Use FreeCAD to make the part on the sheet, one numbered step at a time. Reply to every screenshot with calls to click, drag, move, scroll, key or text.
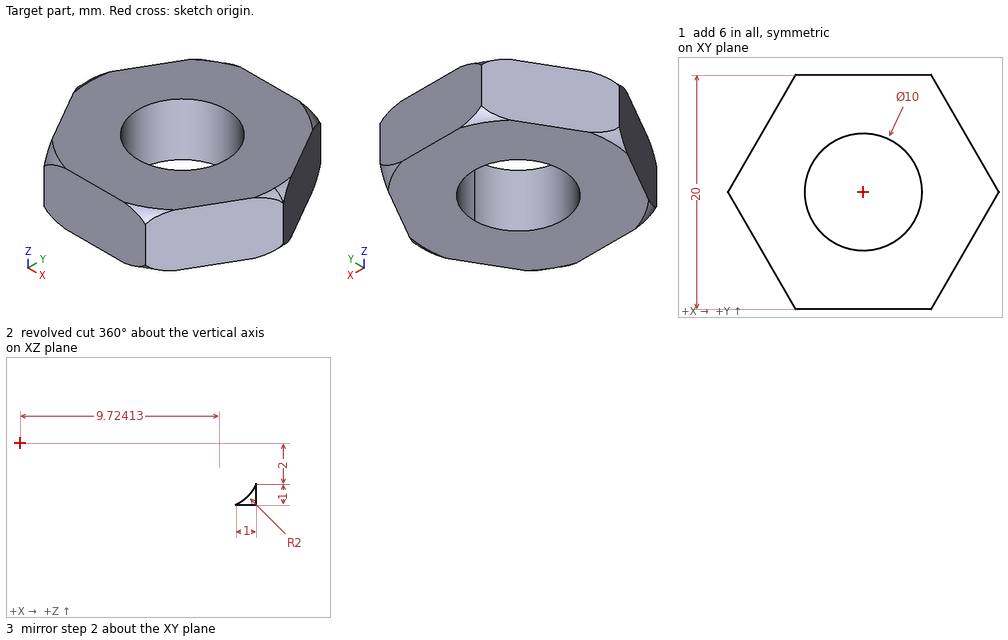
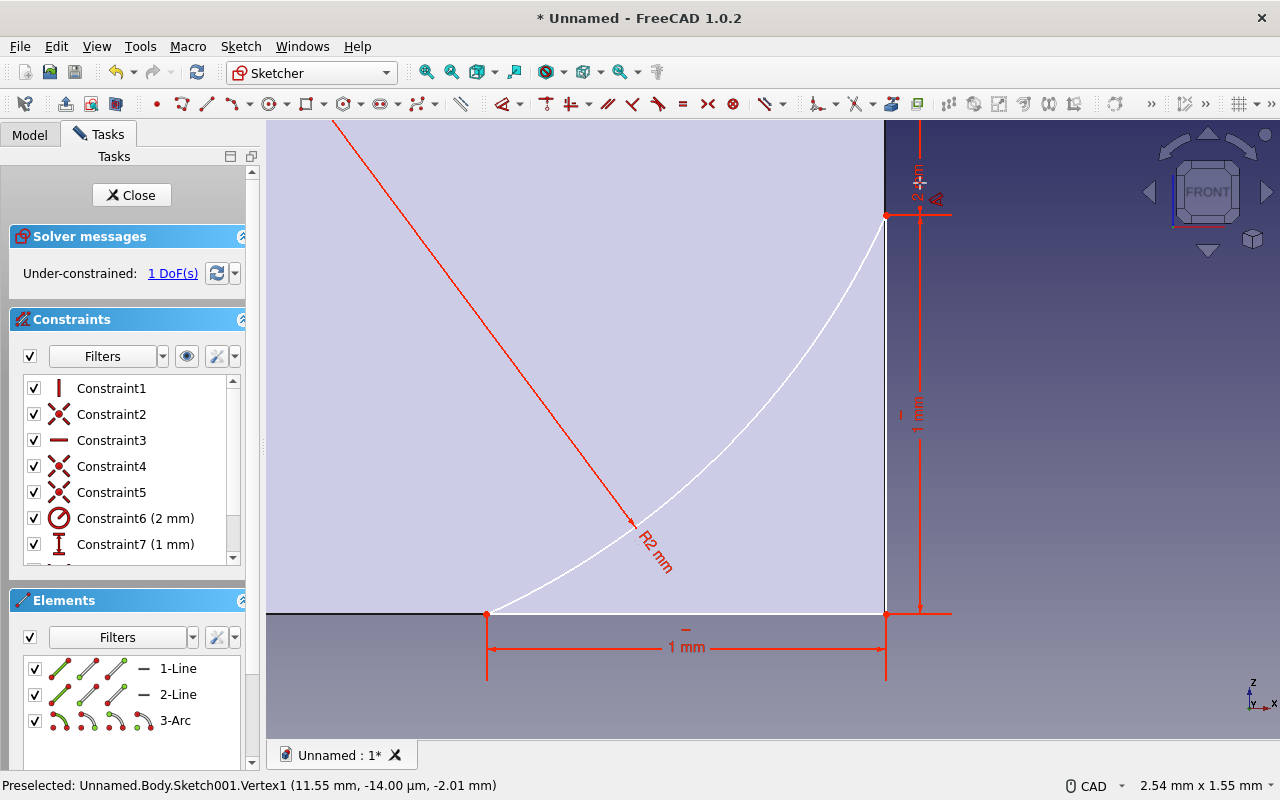
scroll(927, 647, down, 3)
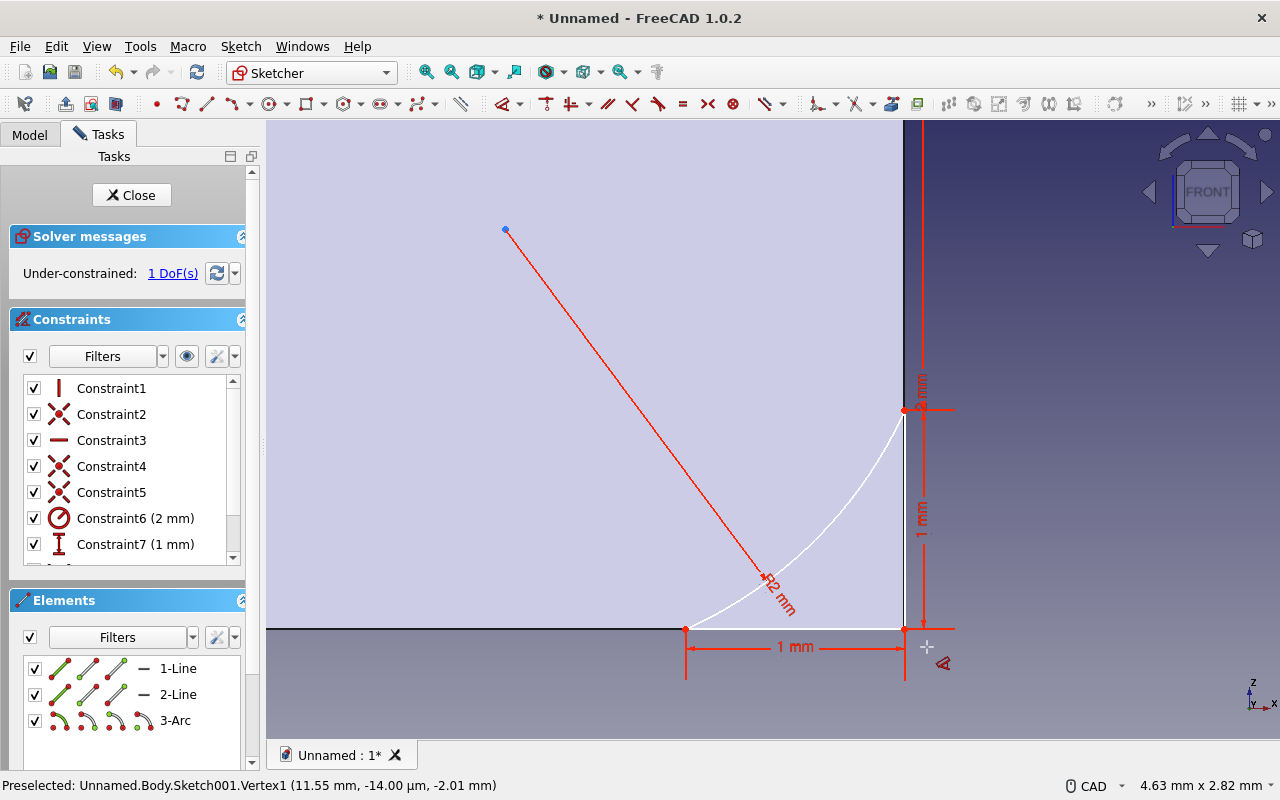
click(505, 230)
click(400, 264)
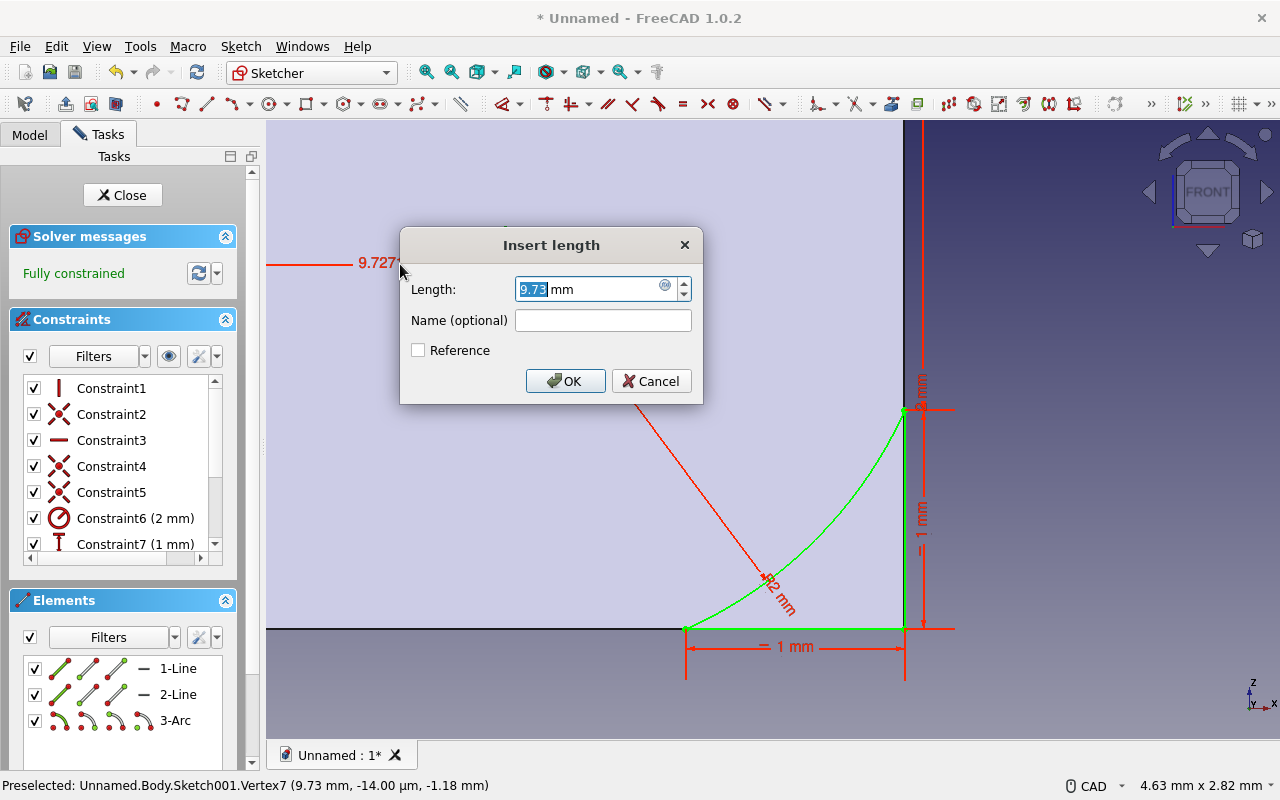
text(9.72413)
key(Return)
key(Escape)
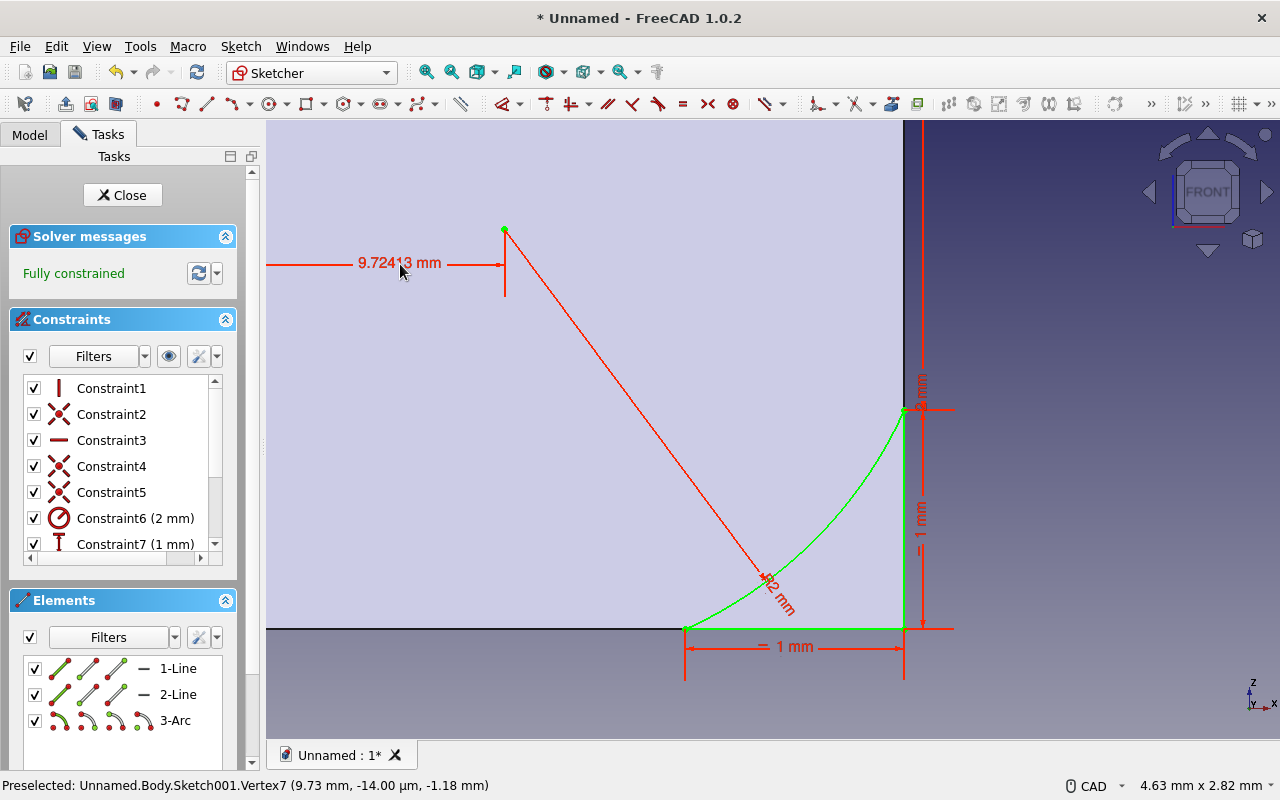
click(123, 195)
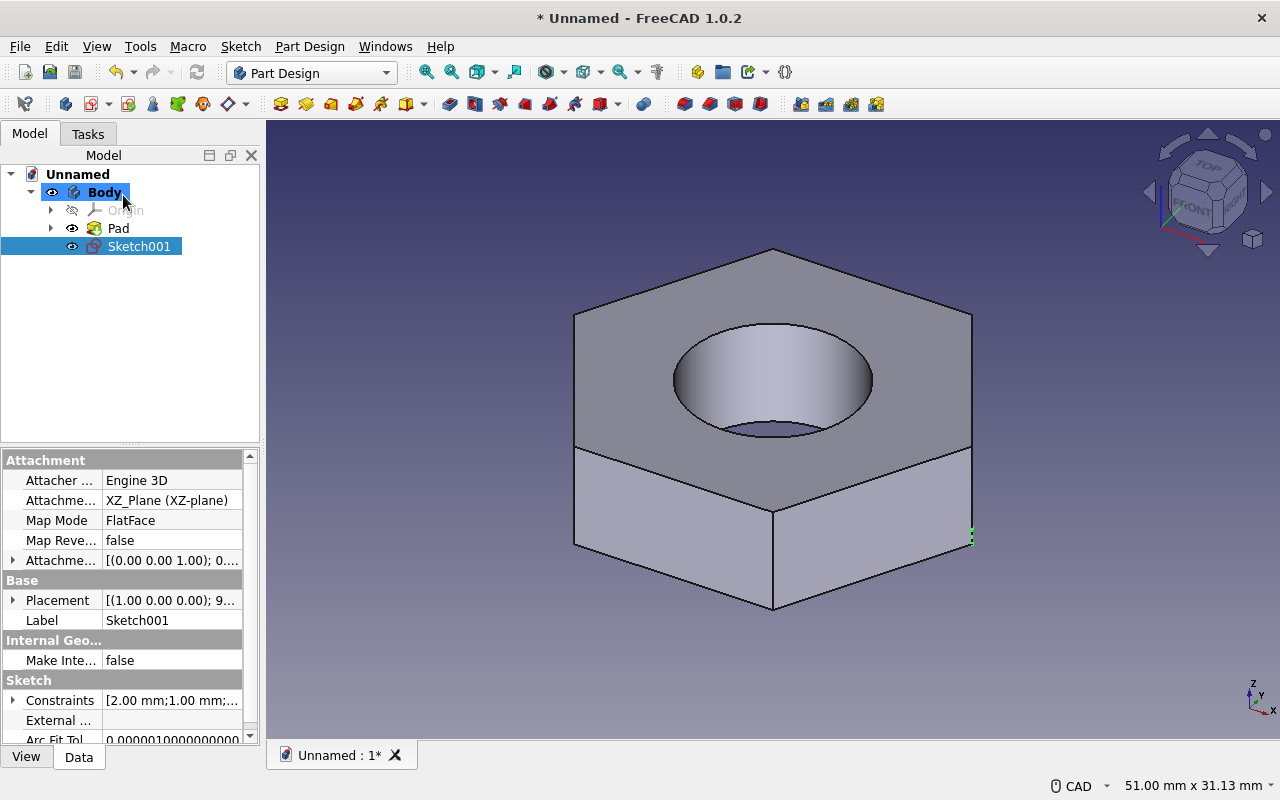
click(500, 104)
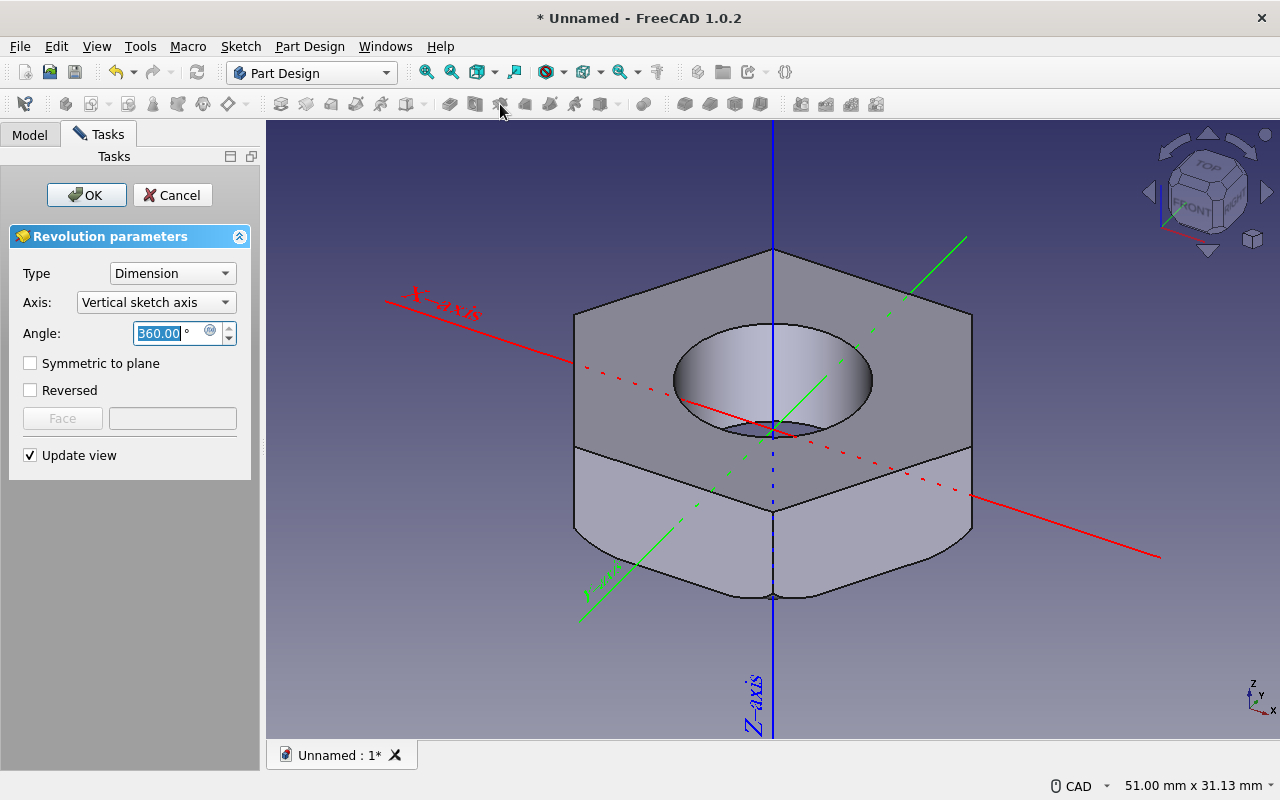
click(87, 195)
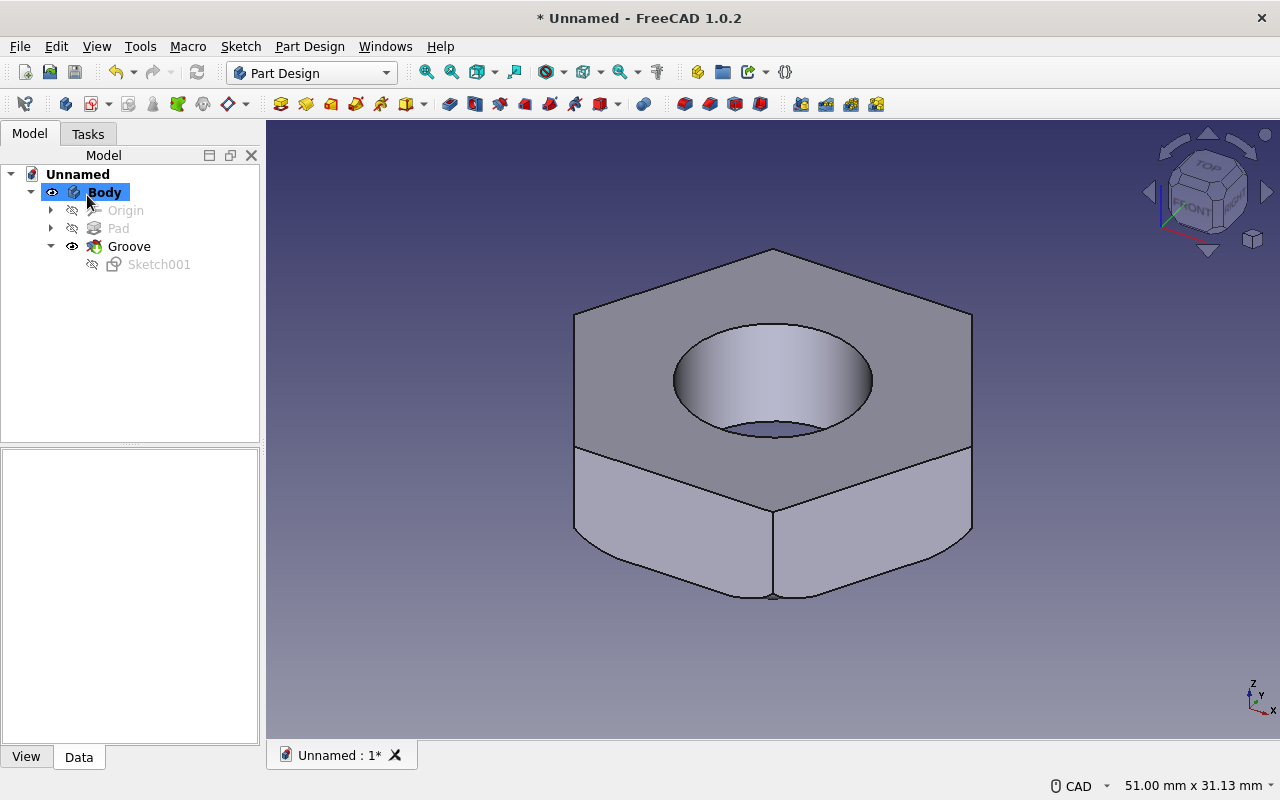
click(117, 246)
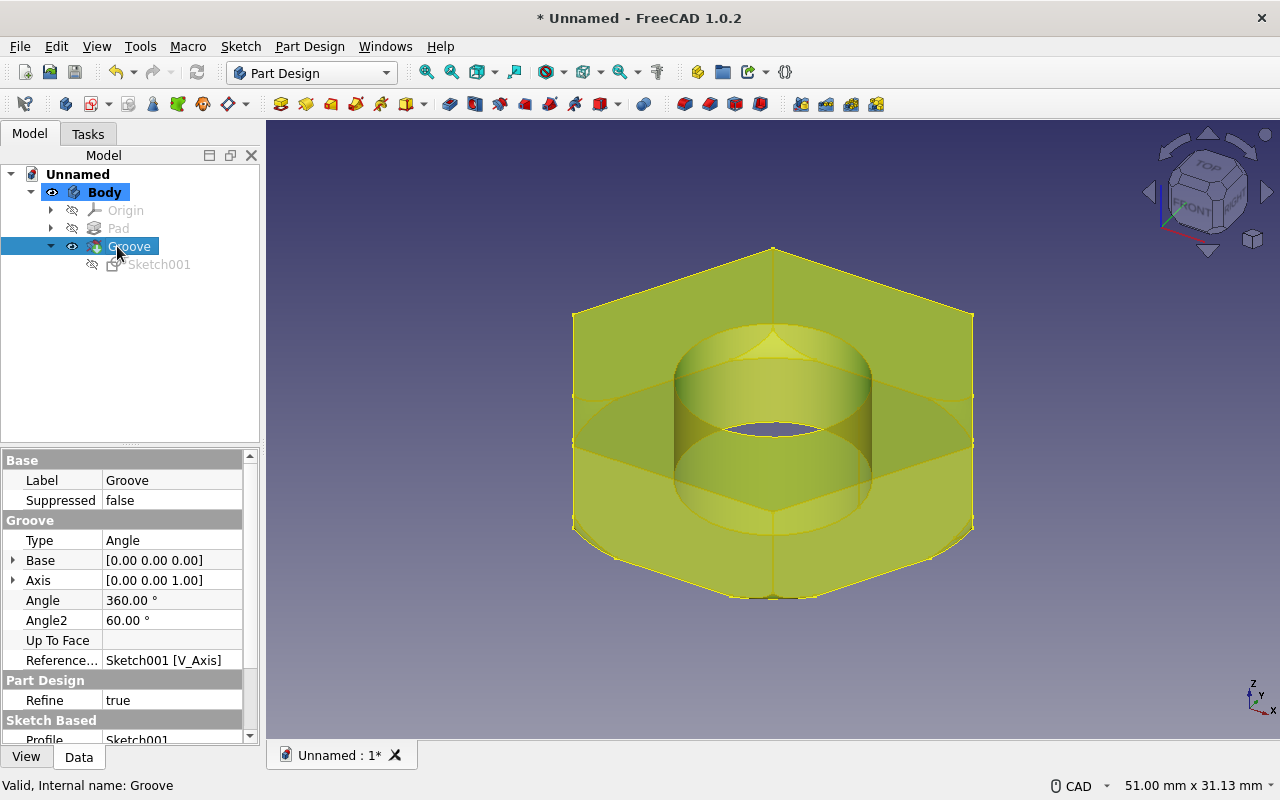
click(801, 104)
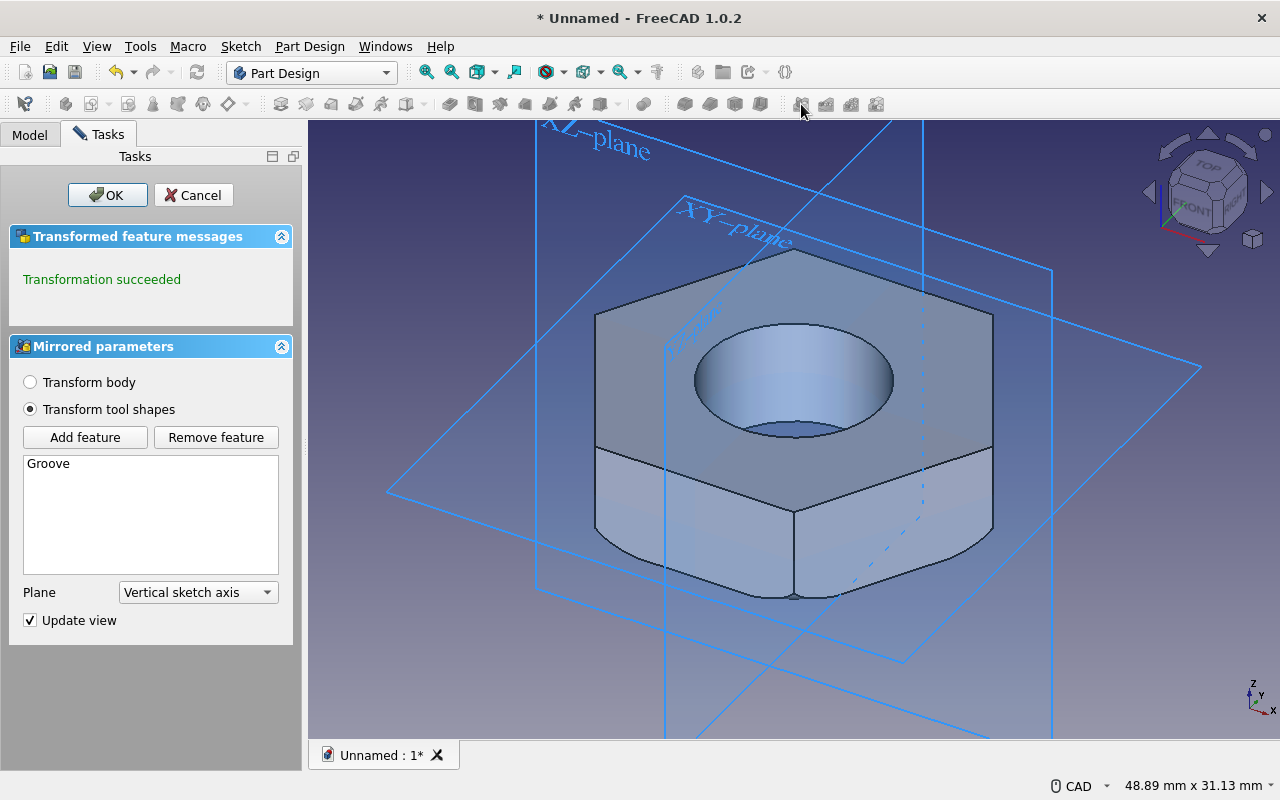
click(199, 592)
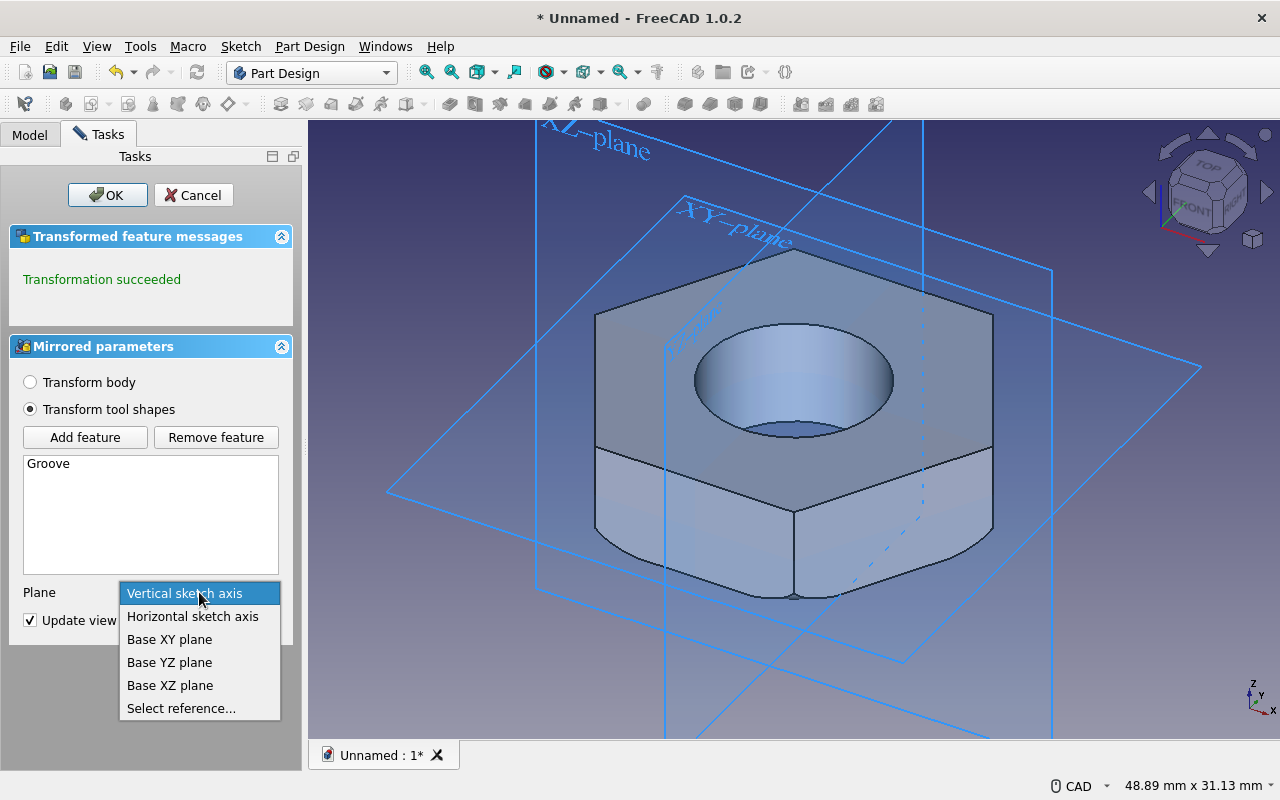
click(198, 640)